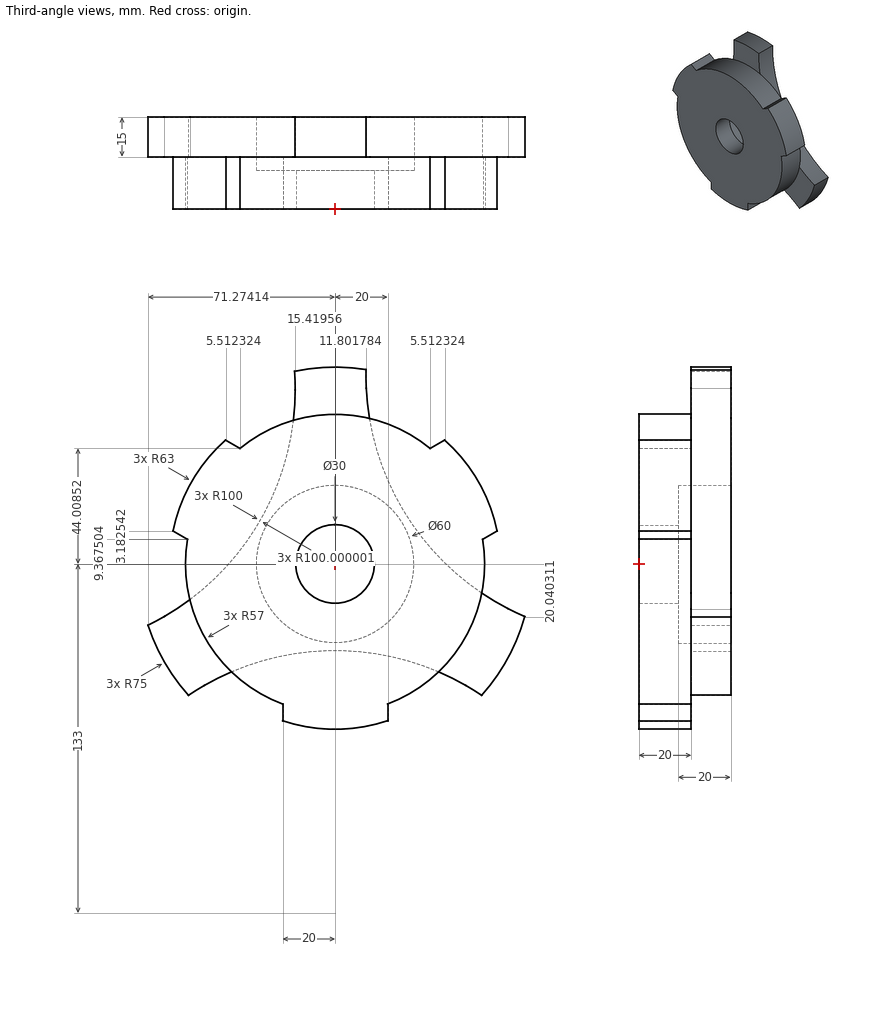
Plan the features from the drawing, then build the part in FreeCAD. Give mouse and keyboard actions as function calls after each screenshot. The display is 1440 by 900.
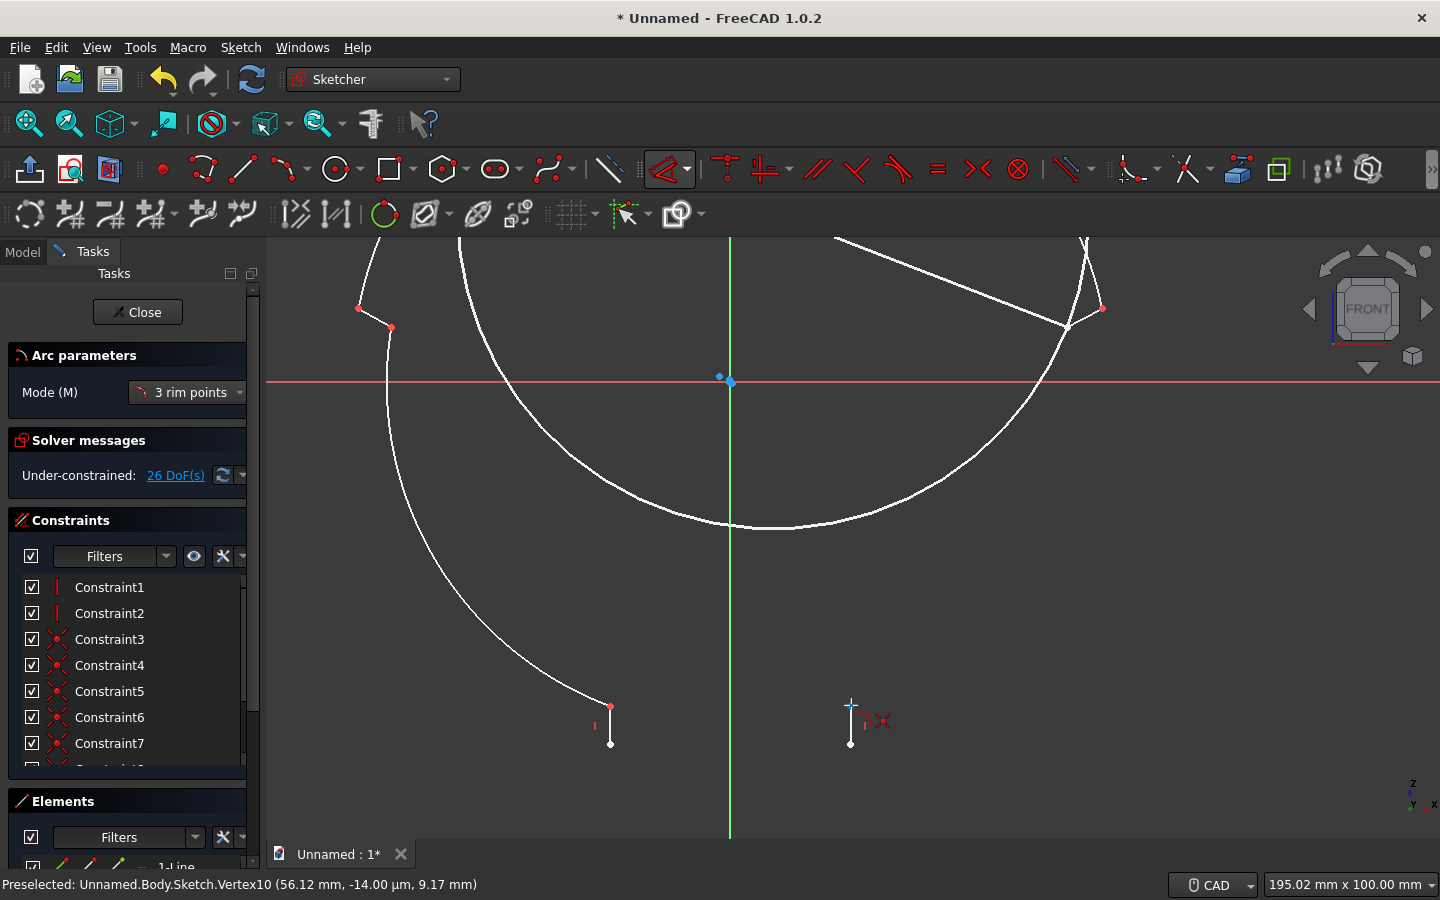
click(851, 706)
click(1027, 554)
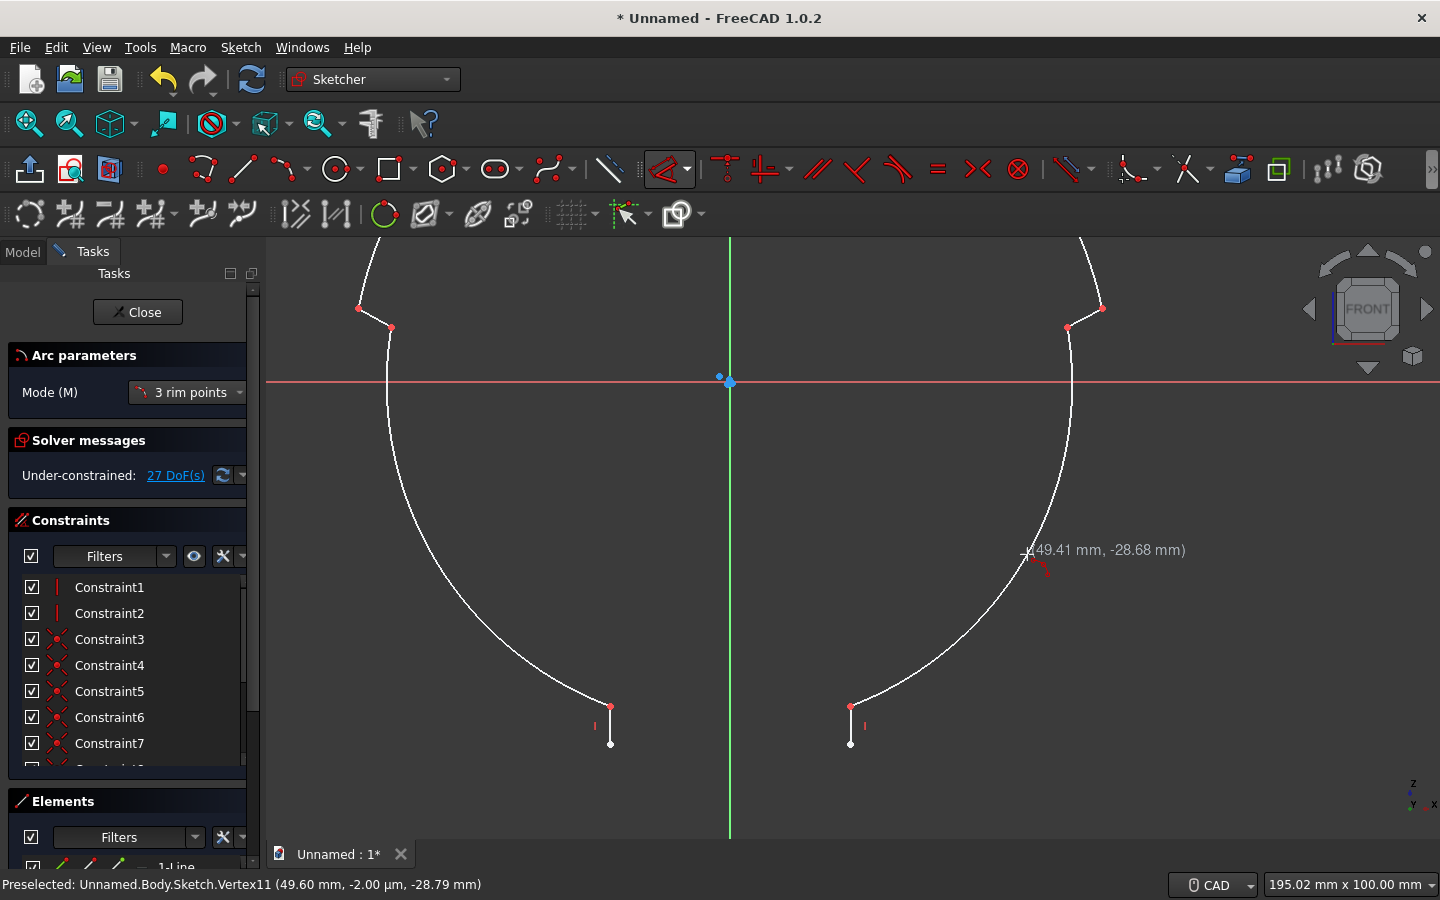
click(851, 744)
click(610, 744)
click(705, 761)
key(Escape)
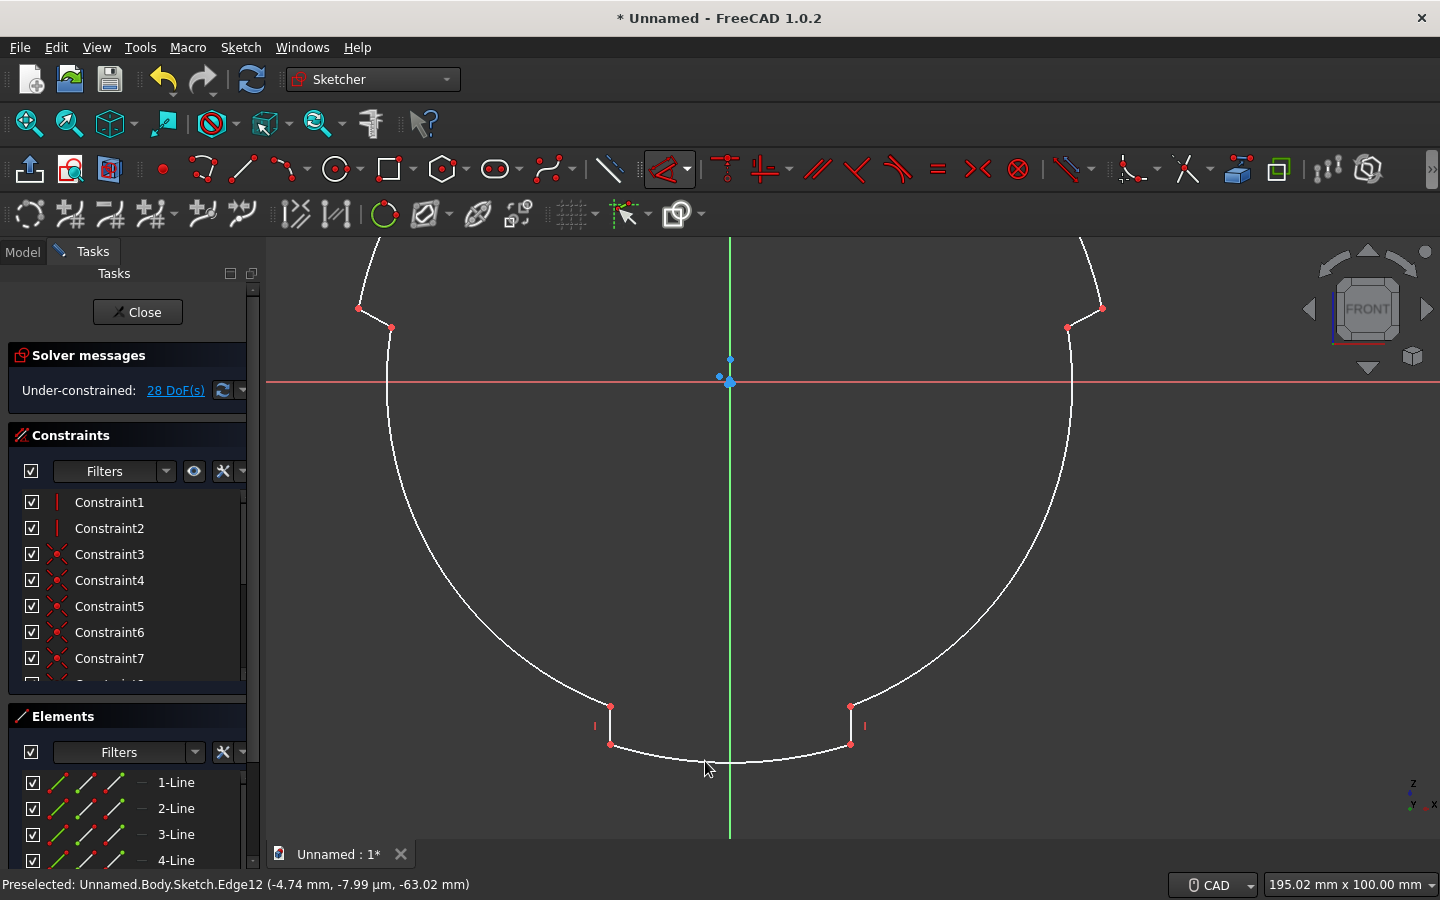
click(397, 468)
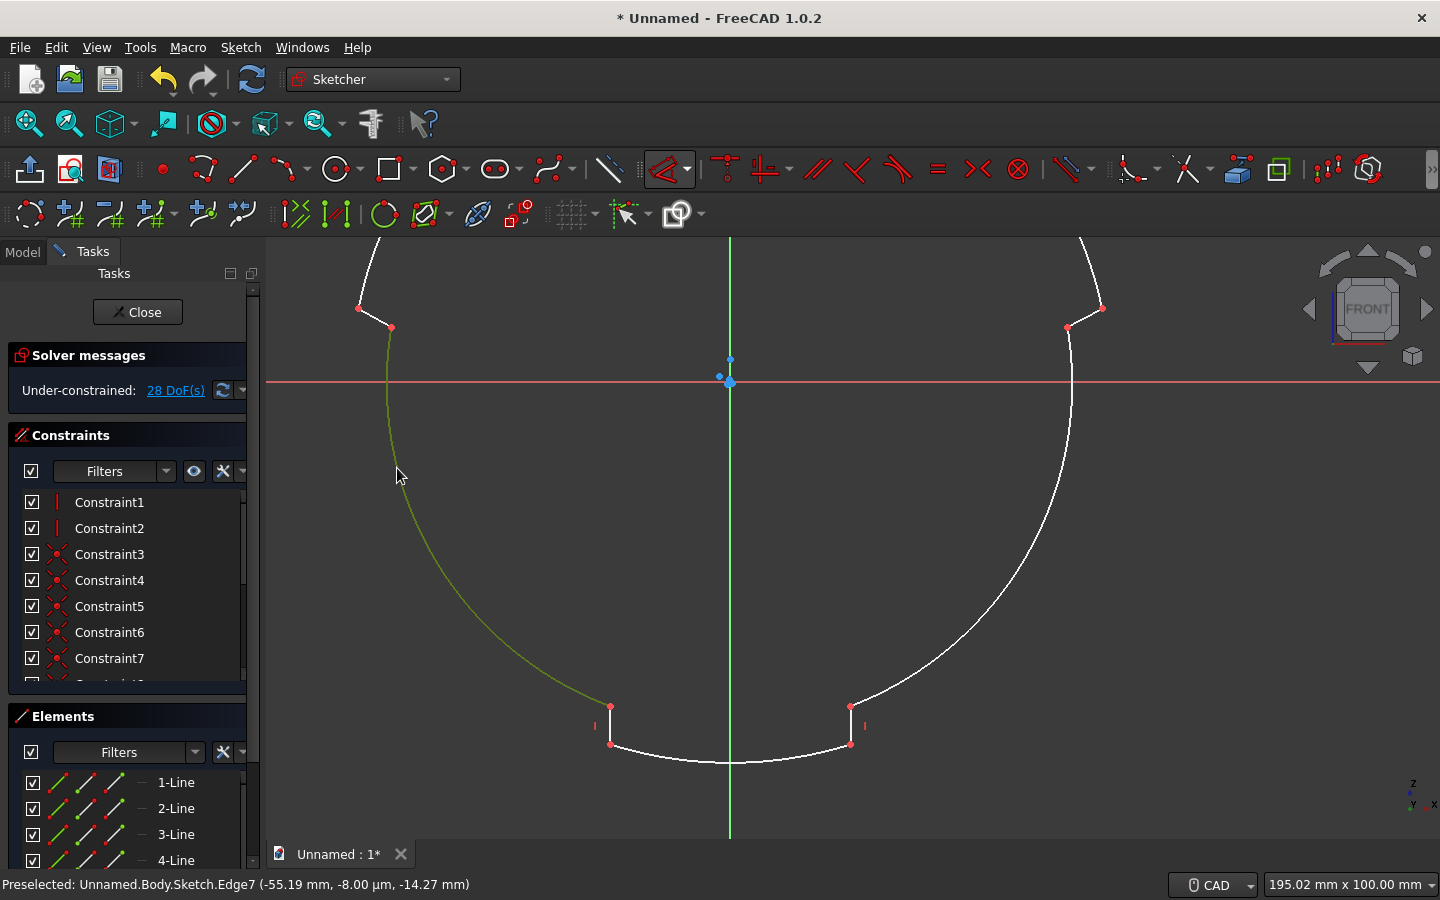
scroll(851, 705, down, 3)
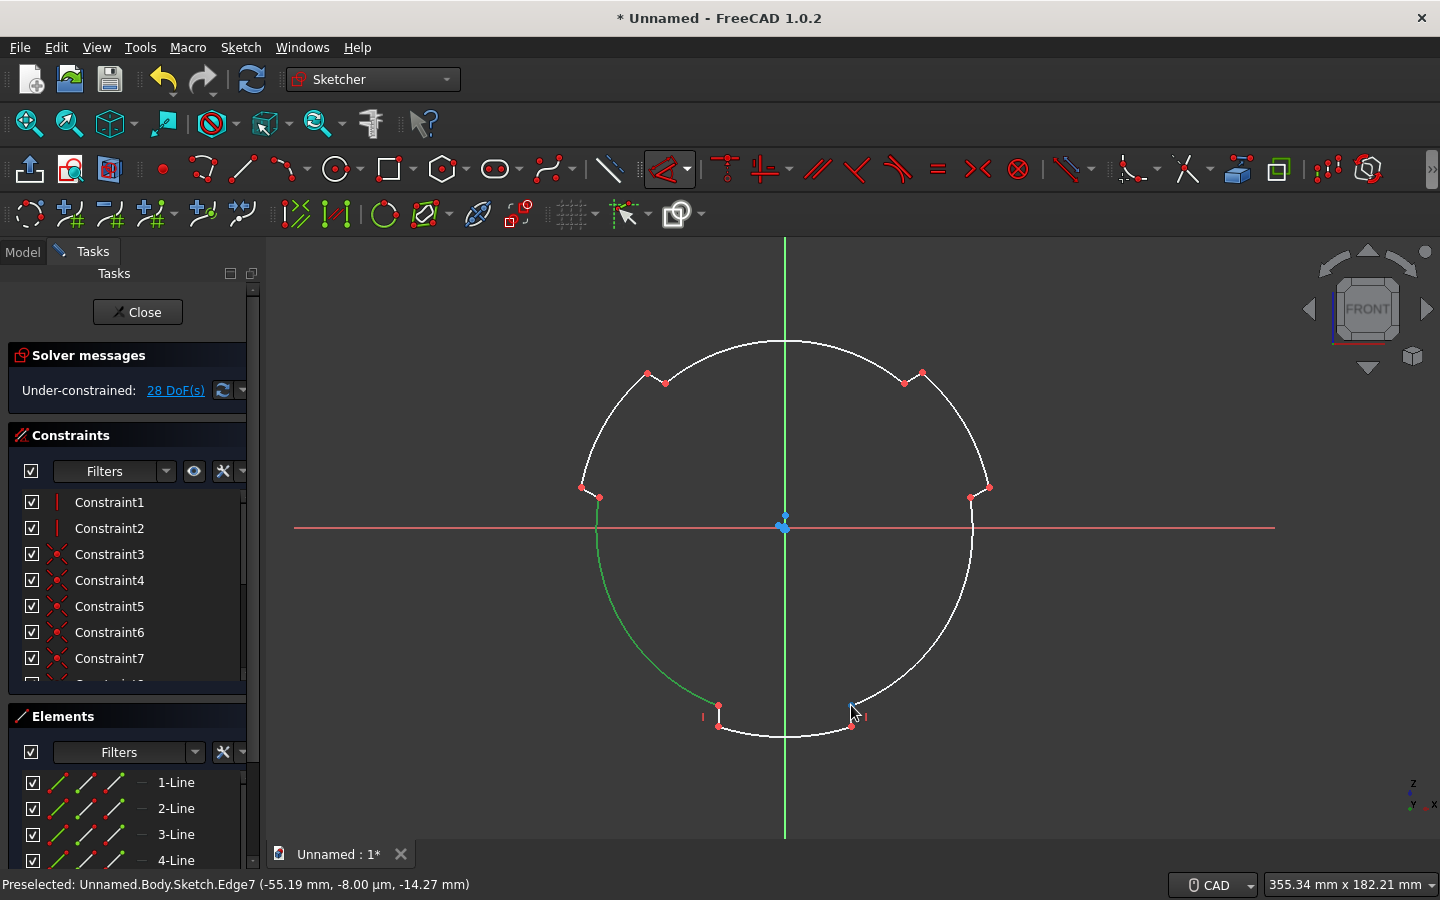
click(619, 402)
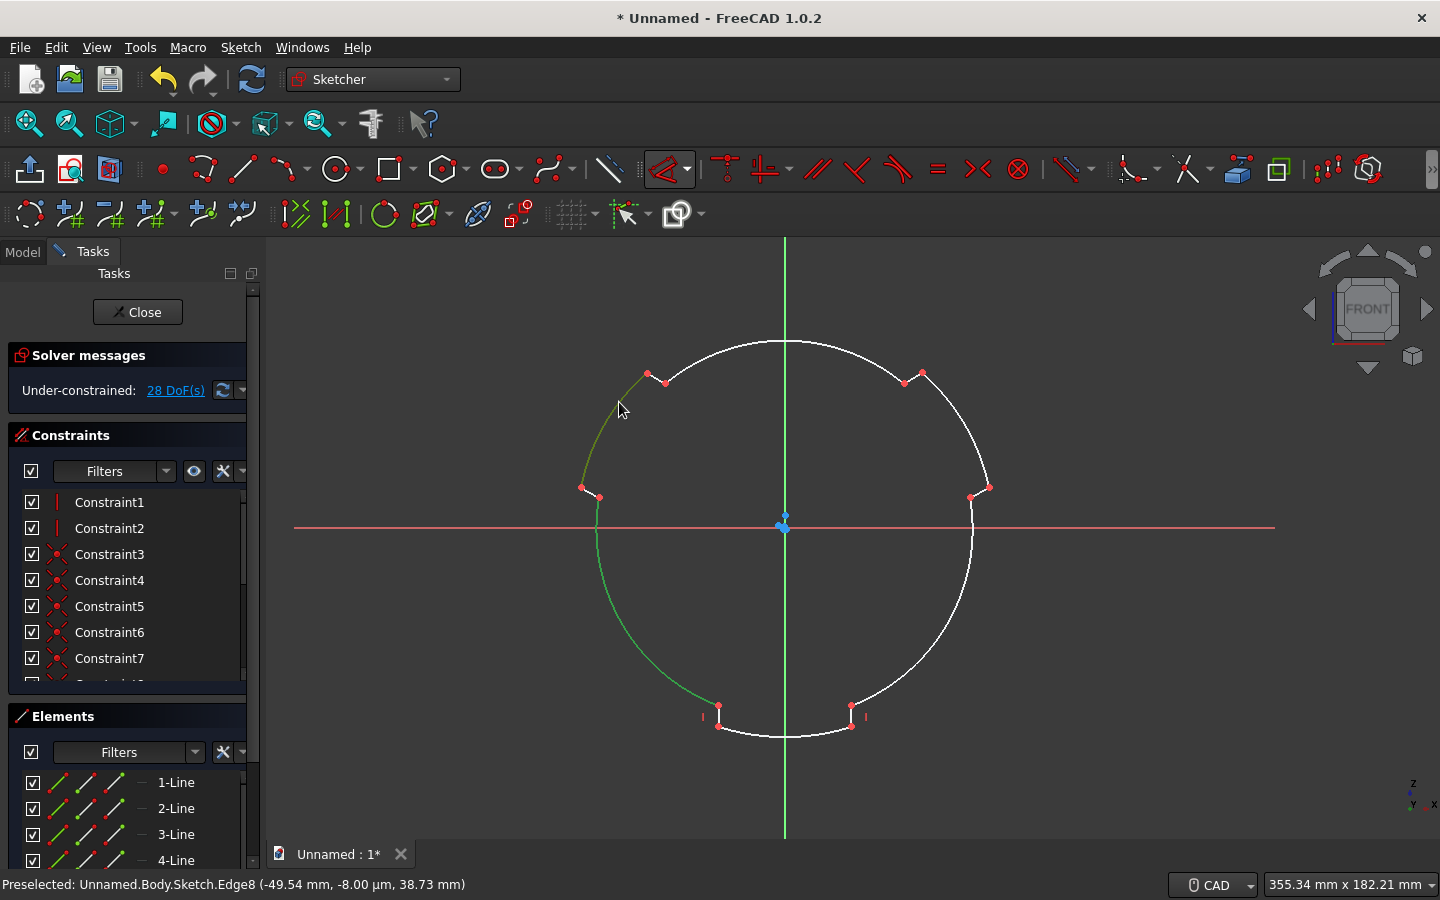
click(726, 170)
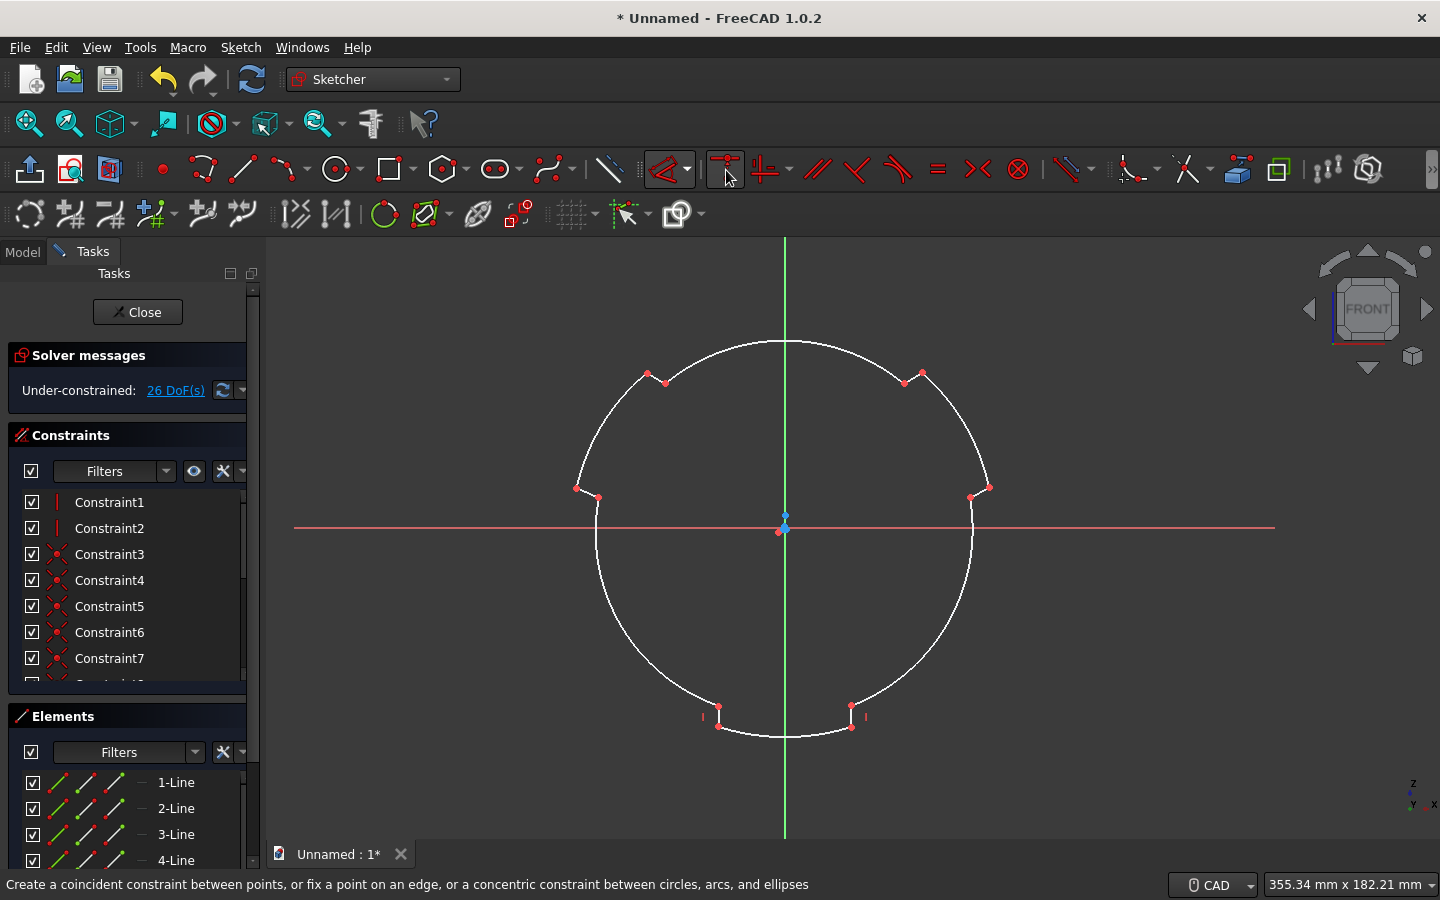
click(601, 576)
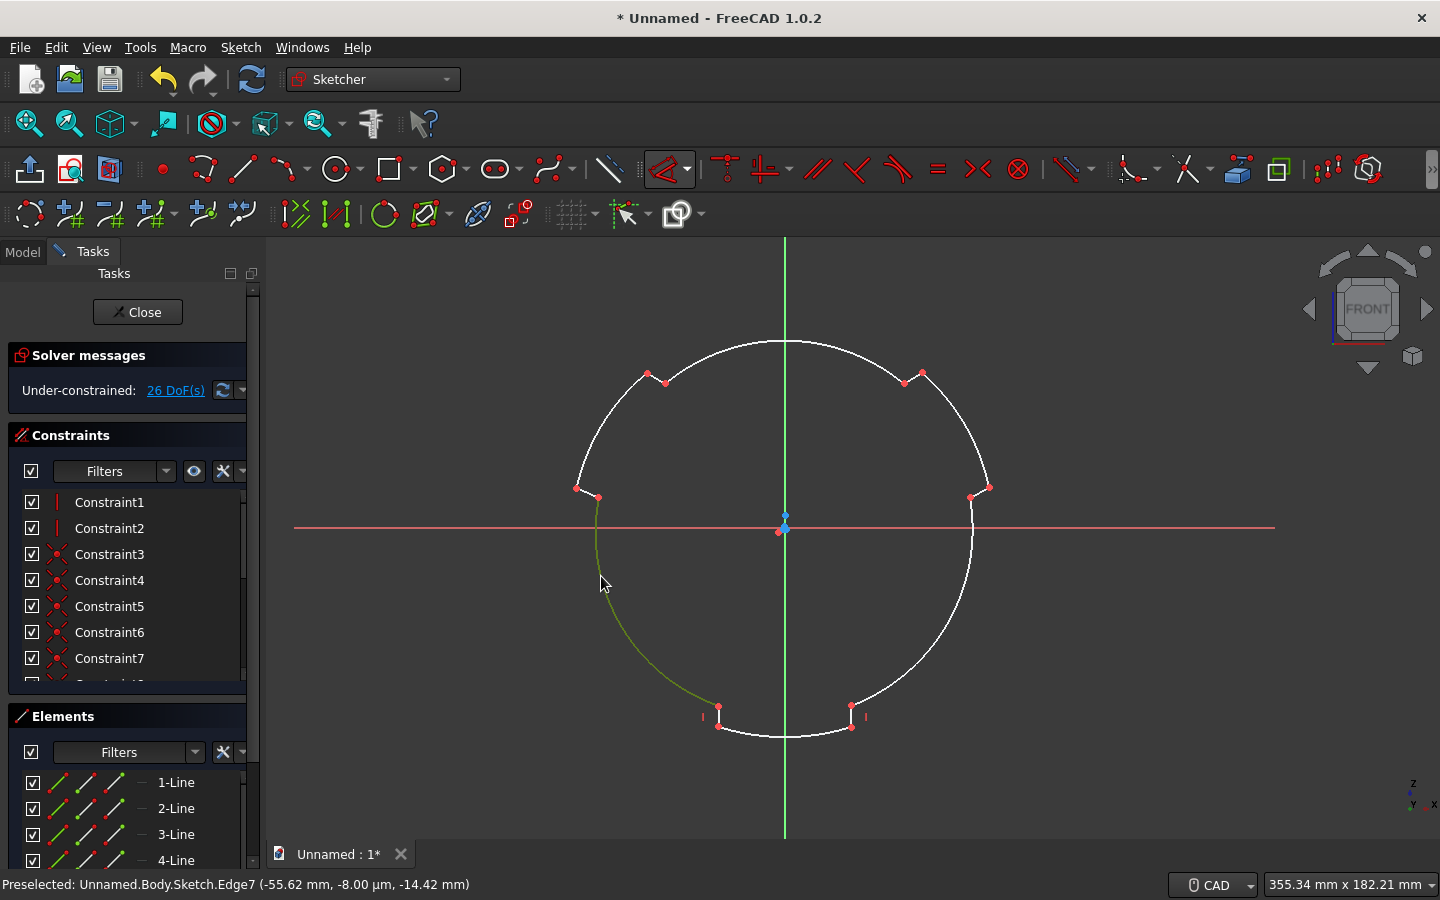
click(836, 348)